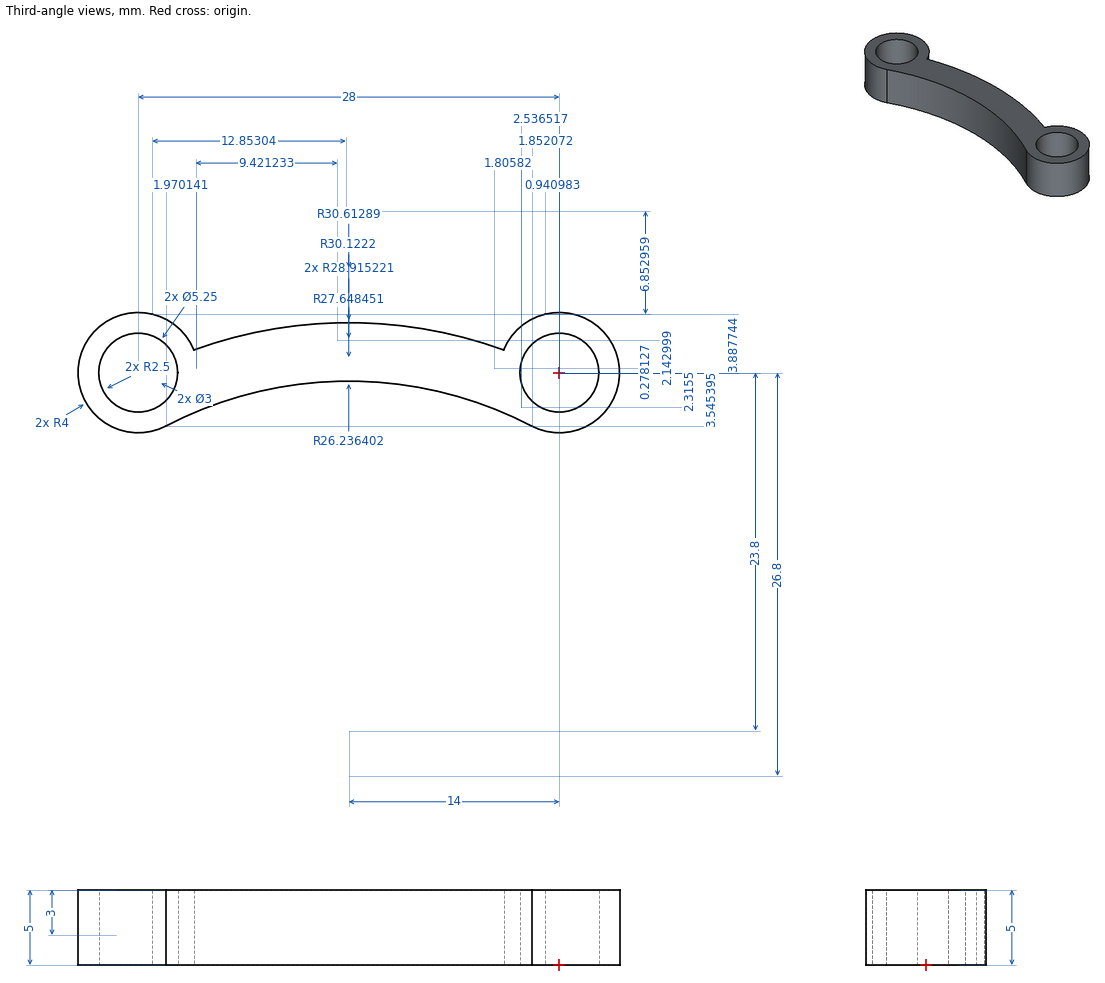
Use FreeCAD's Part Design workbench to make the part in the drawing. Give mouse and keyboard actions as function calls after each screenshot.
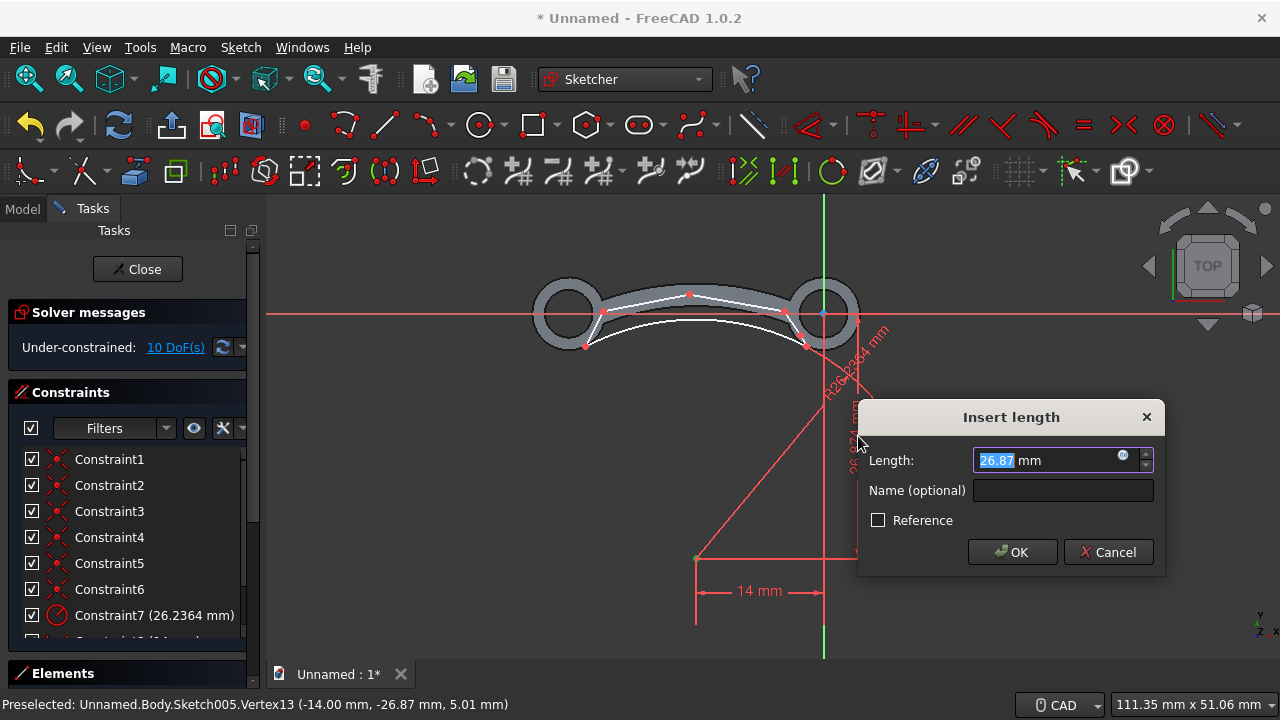
text(26.8)
key(Return)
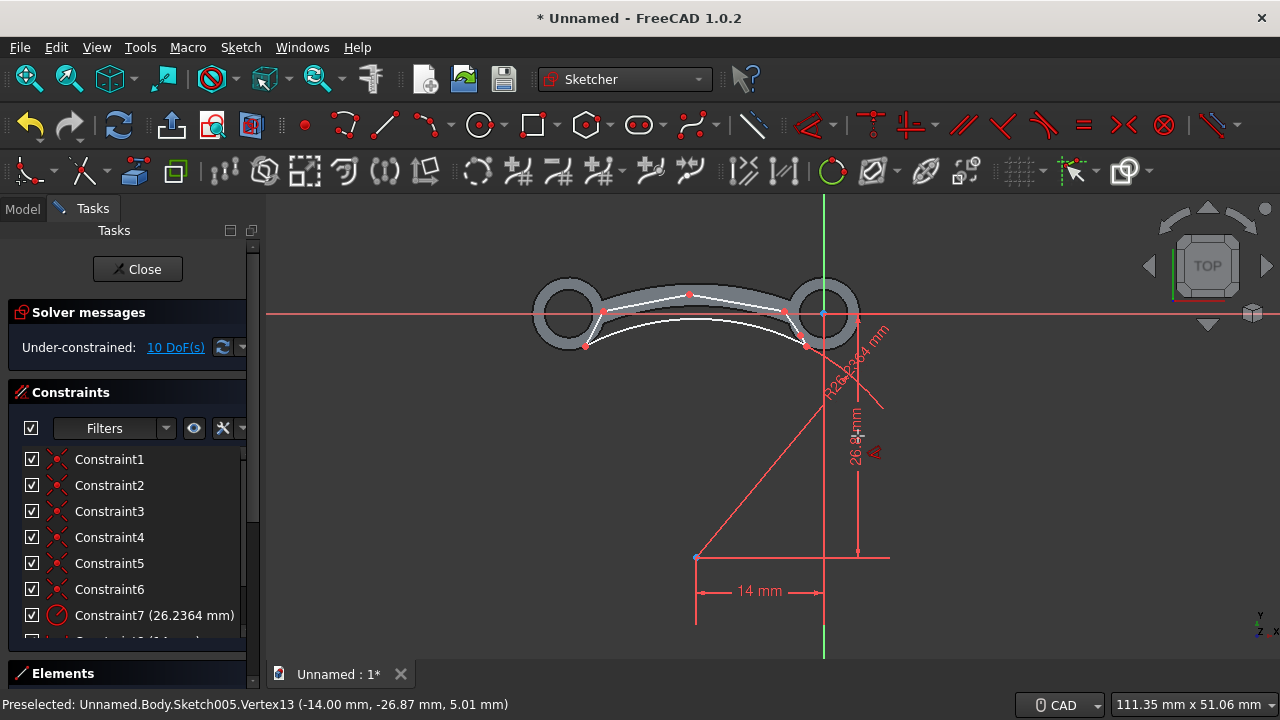
scroll(801, 335, up, 4)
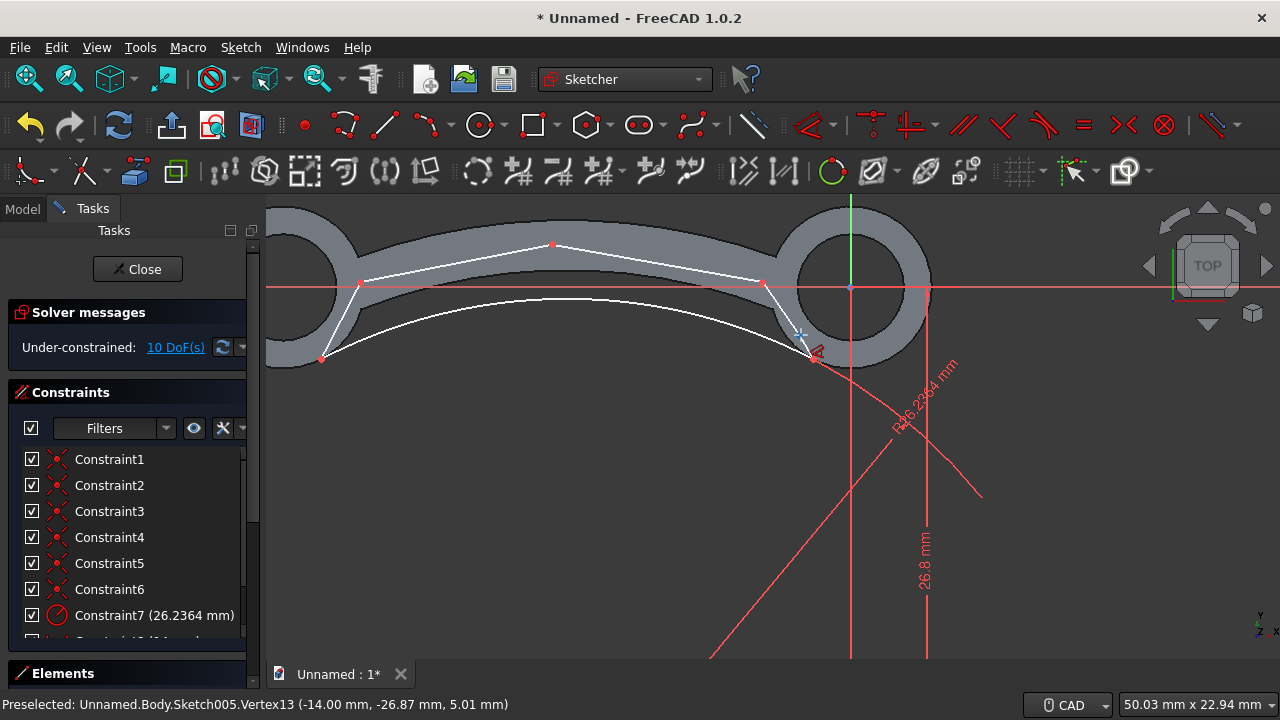
click(800, 335)
click(885, 311)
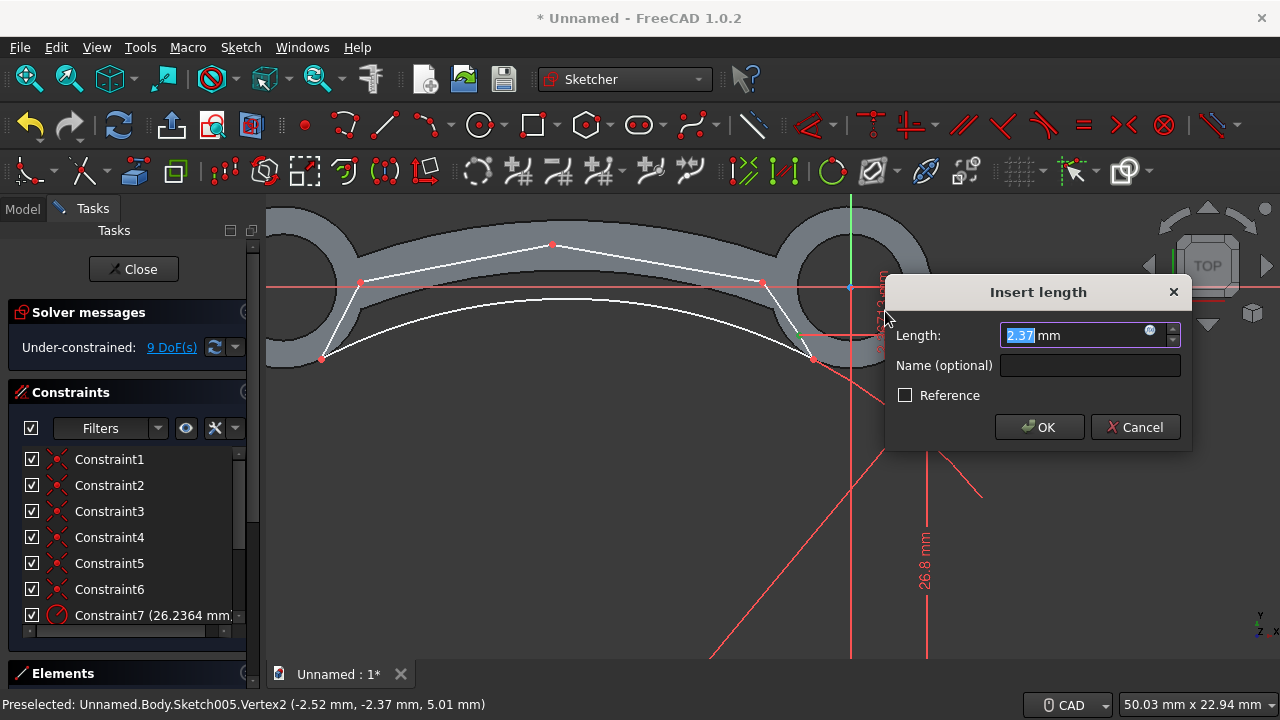
text(2.3155)
key(Return)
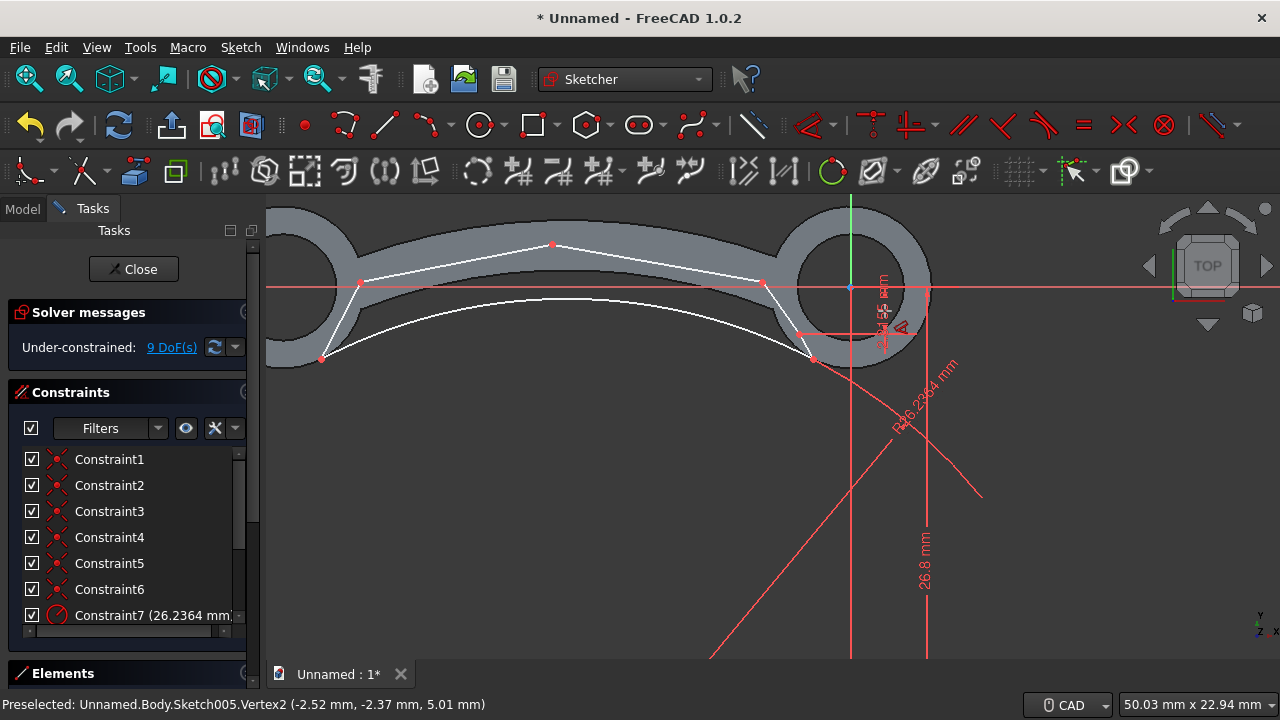
click(789, 319)
click(781, 368)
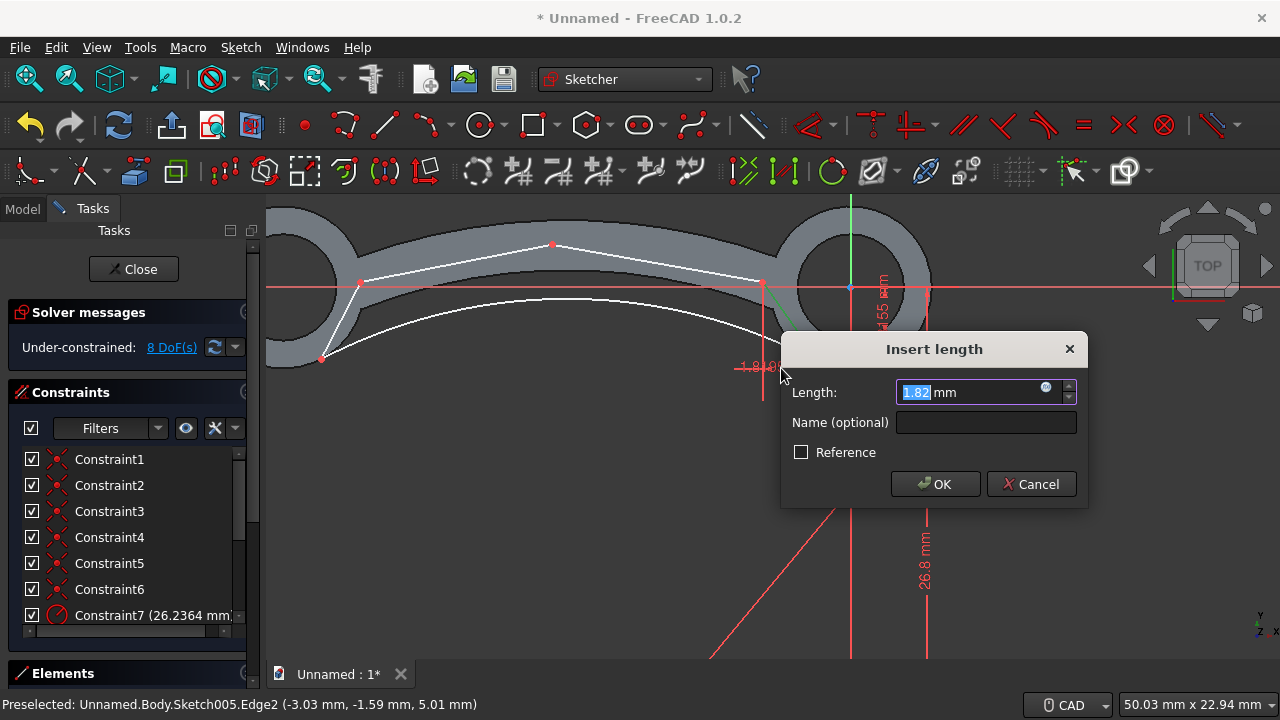
text(1.80582)
key(Return)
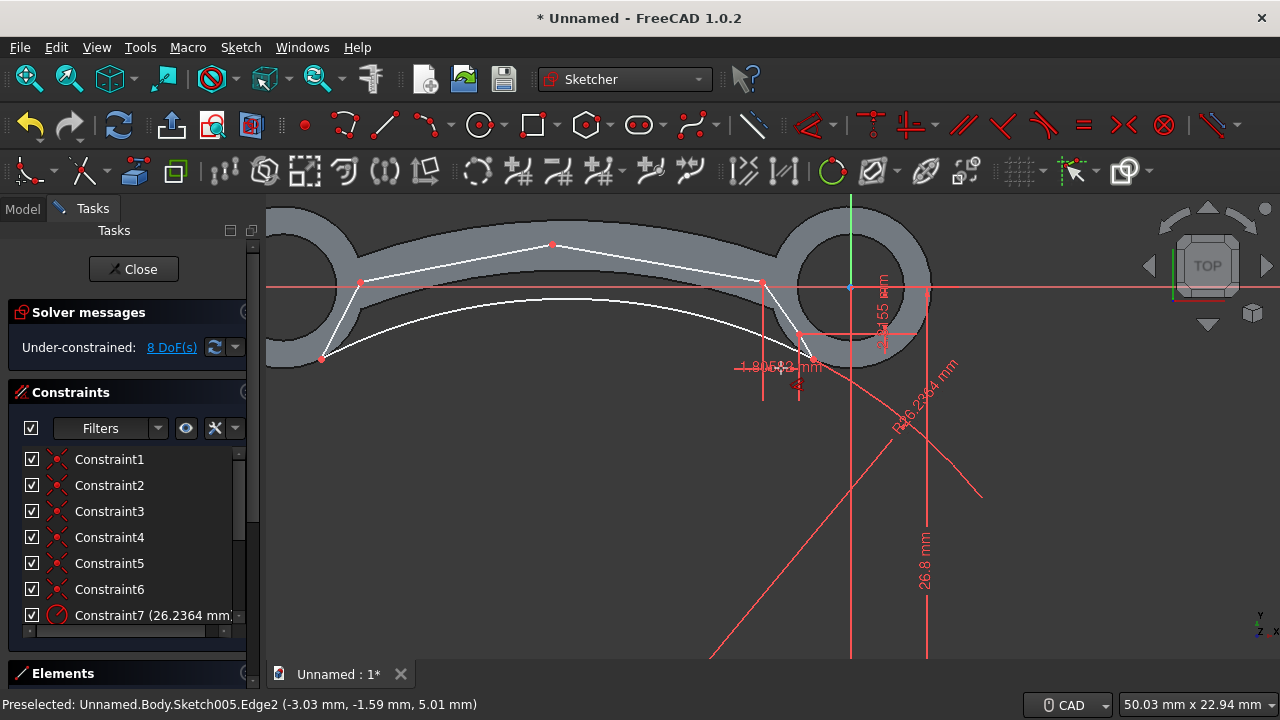
click(814, 360)
click(832, 394)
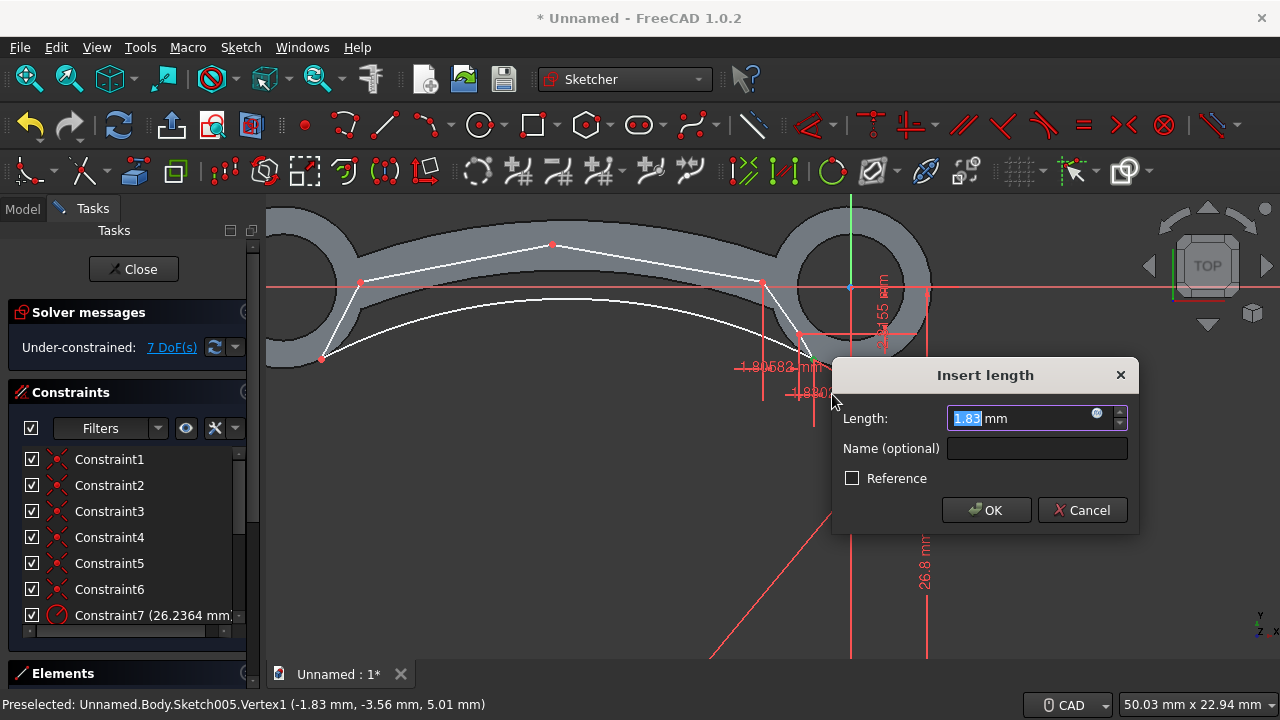
text(1.852072)
key(Return)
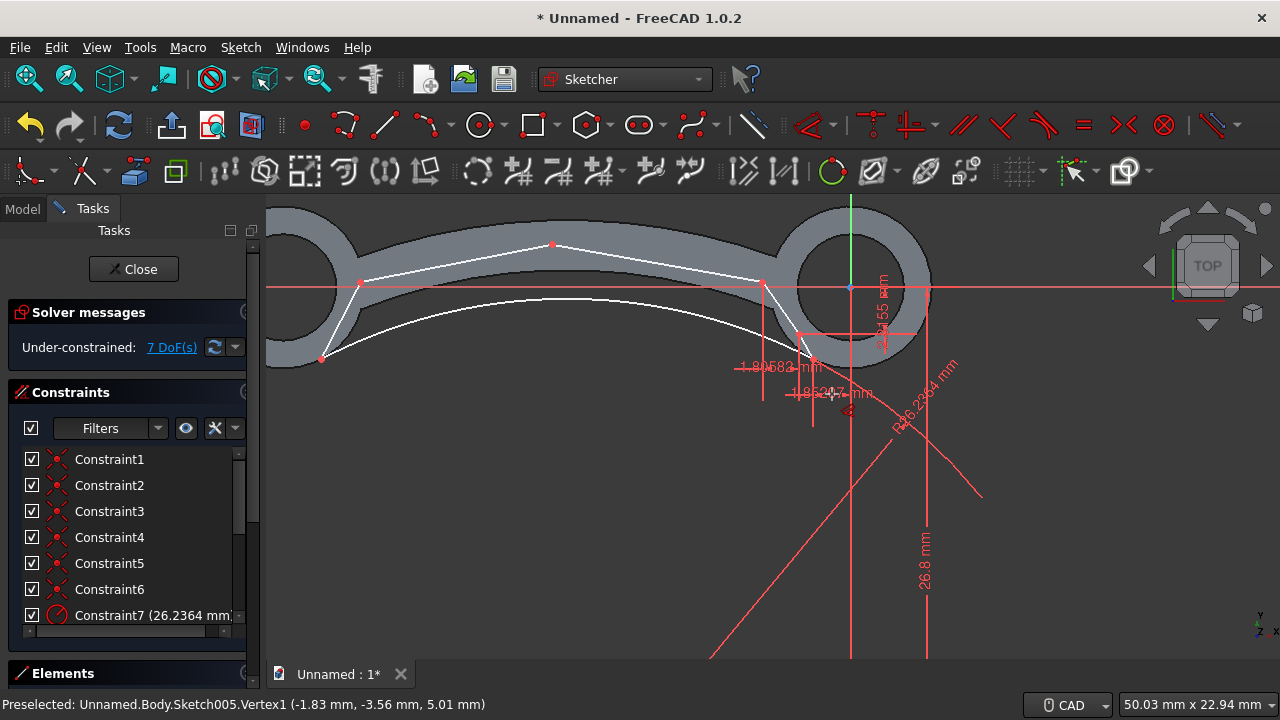
click(799, 334)
click(825, 253)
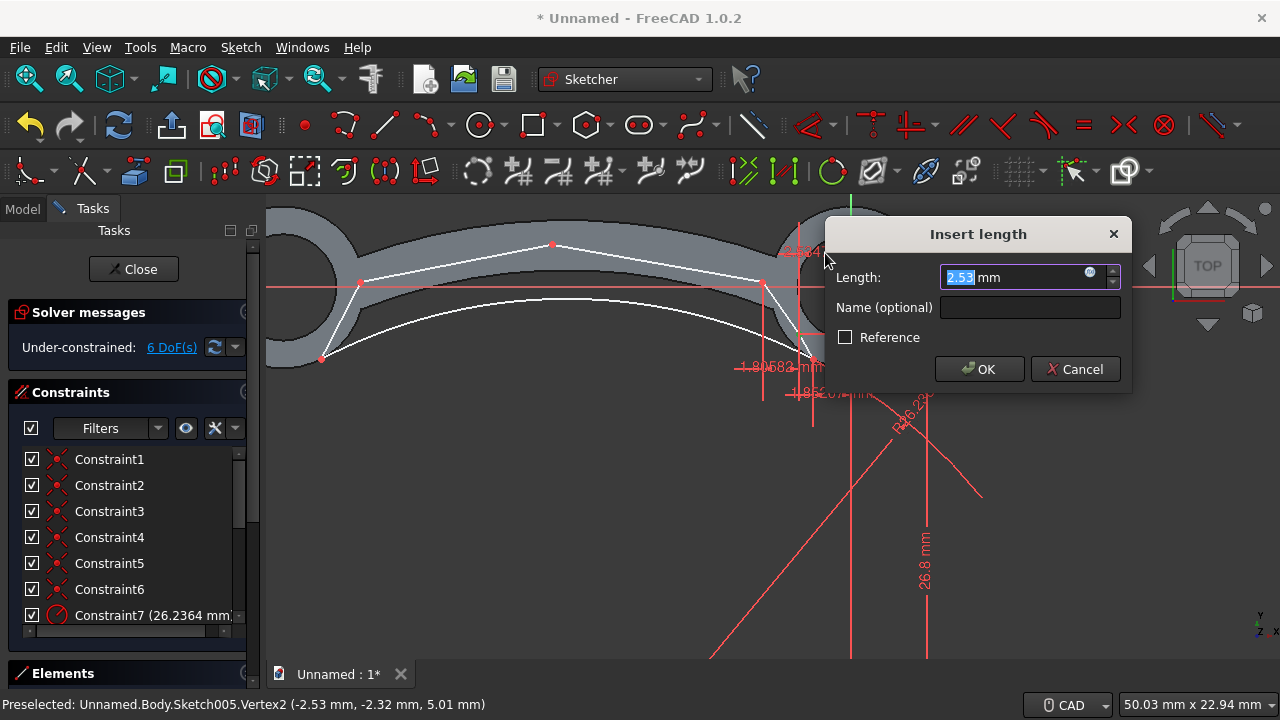
text(2.536517)
key(Return)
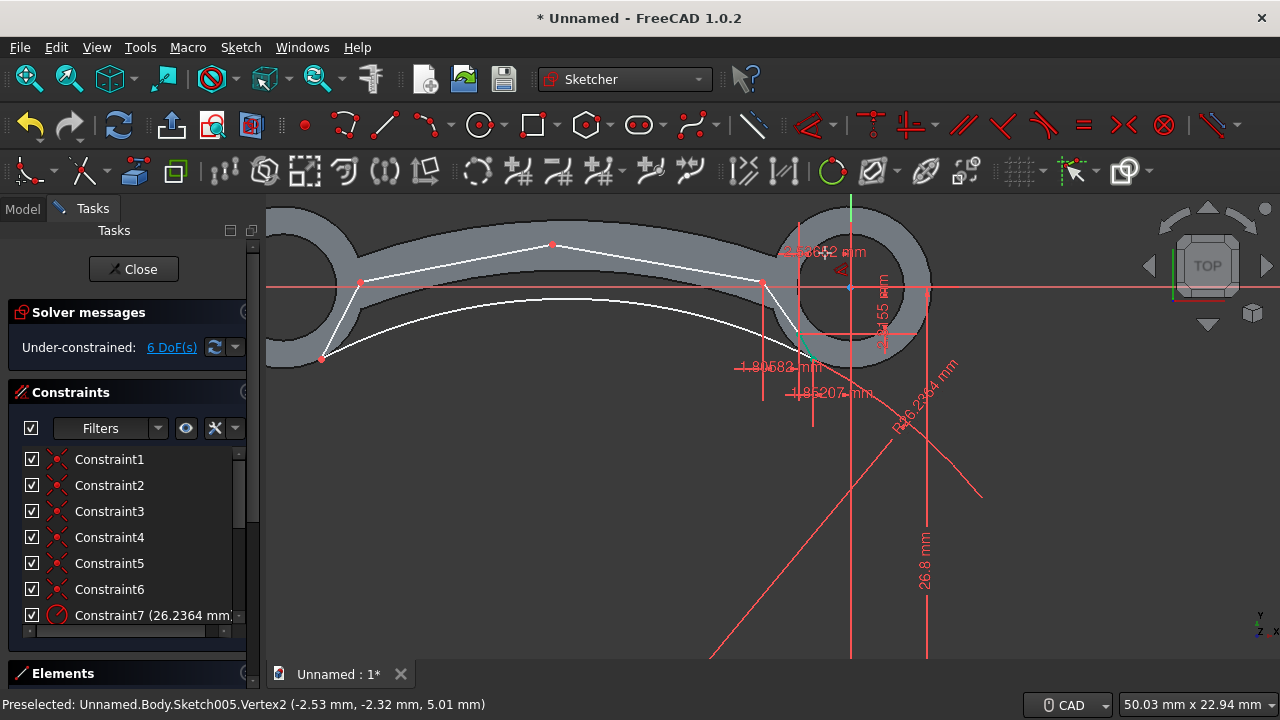
scroll(763, 282, up, 10)